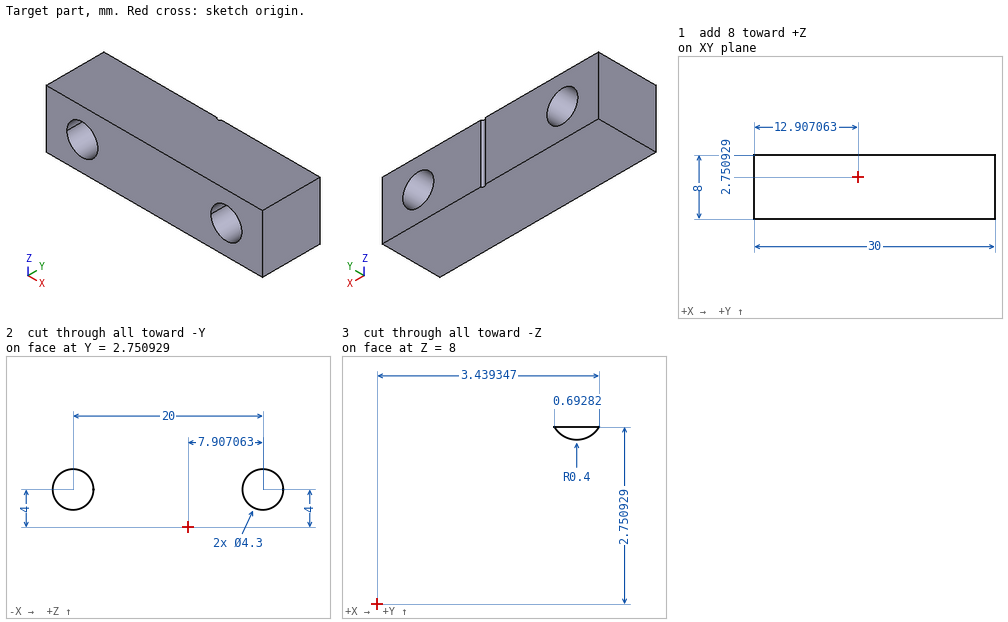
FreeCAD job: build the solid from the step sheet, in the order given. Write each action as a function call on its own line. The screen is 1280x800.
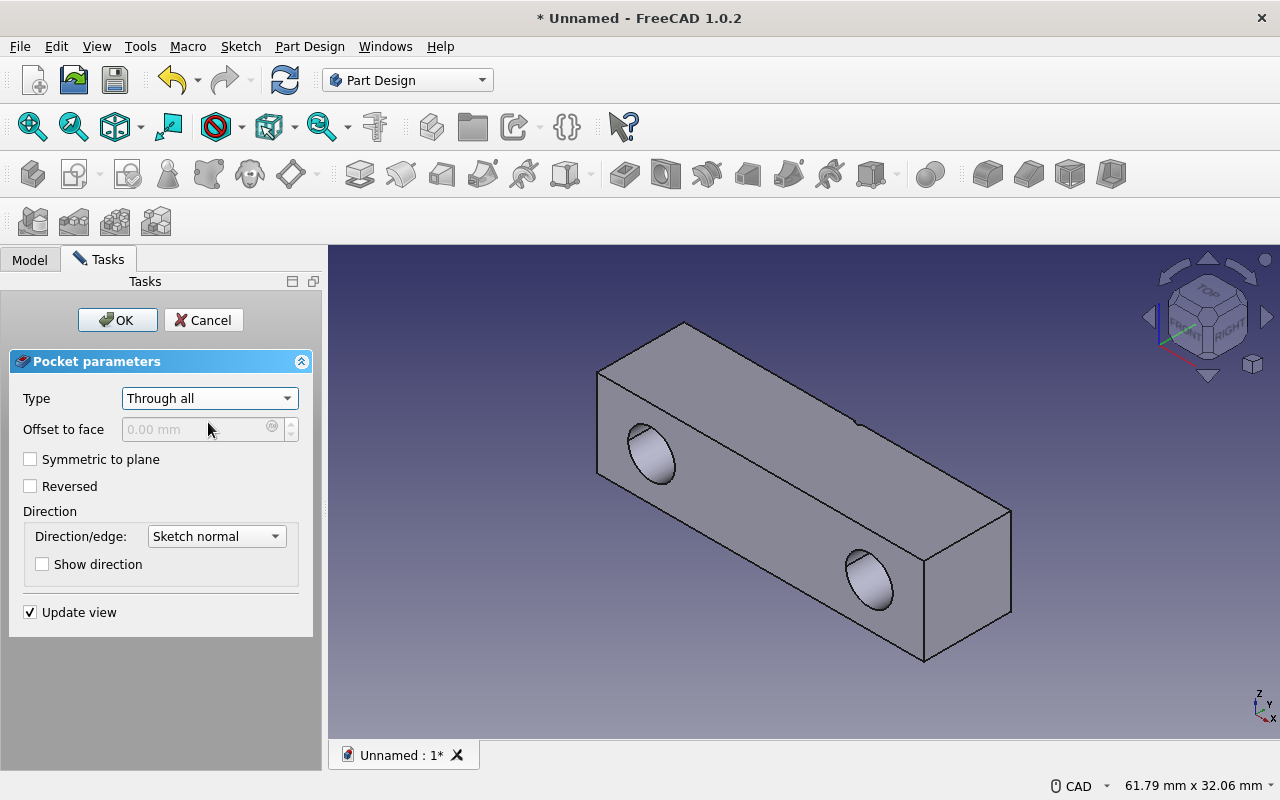
click(118, 320)